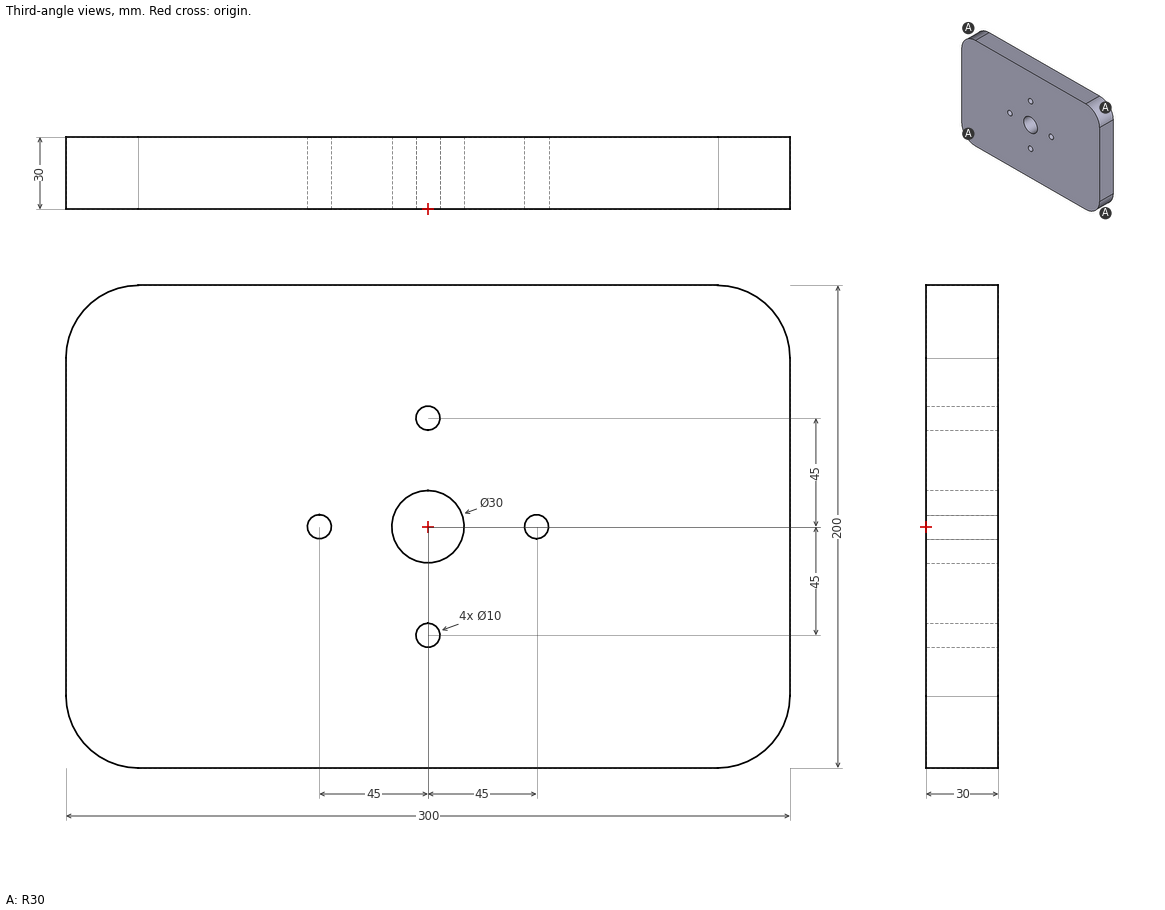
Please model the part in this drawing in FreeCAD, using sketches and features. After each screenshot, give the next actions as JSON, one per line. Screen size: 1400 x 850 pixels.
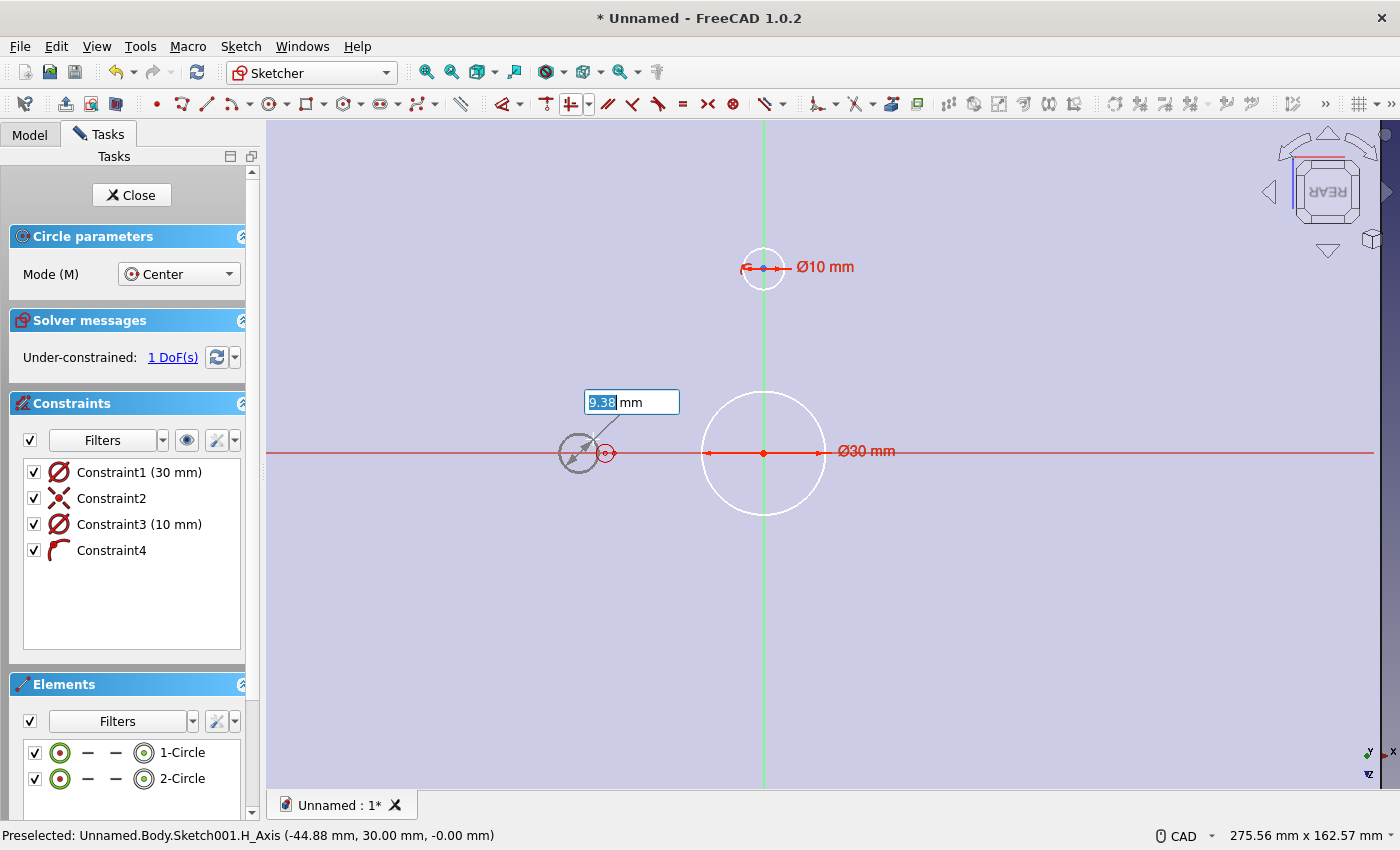
{"action": "type", "text": "10"}
{"action": "key", "text": "Return"}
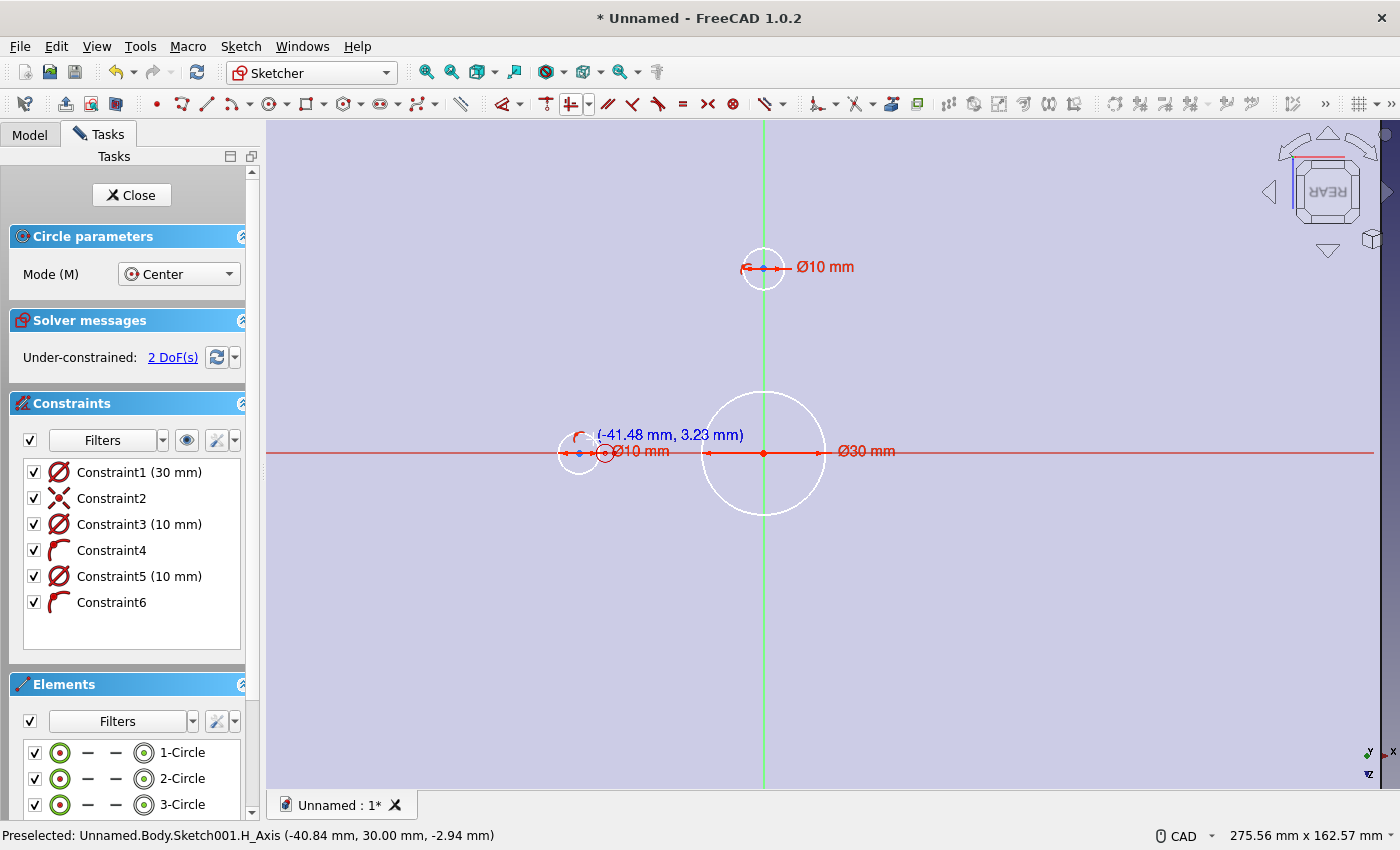
{"action": "left_click", "coordinate": [764, 638]}
{"action": "mouse_move", "coordinate": [778, 624]}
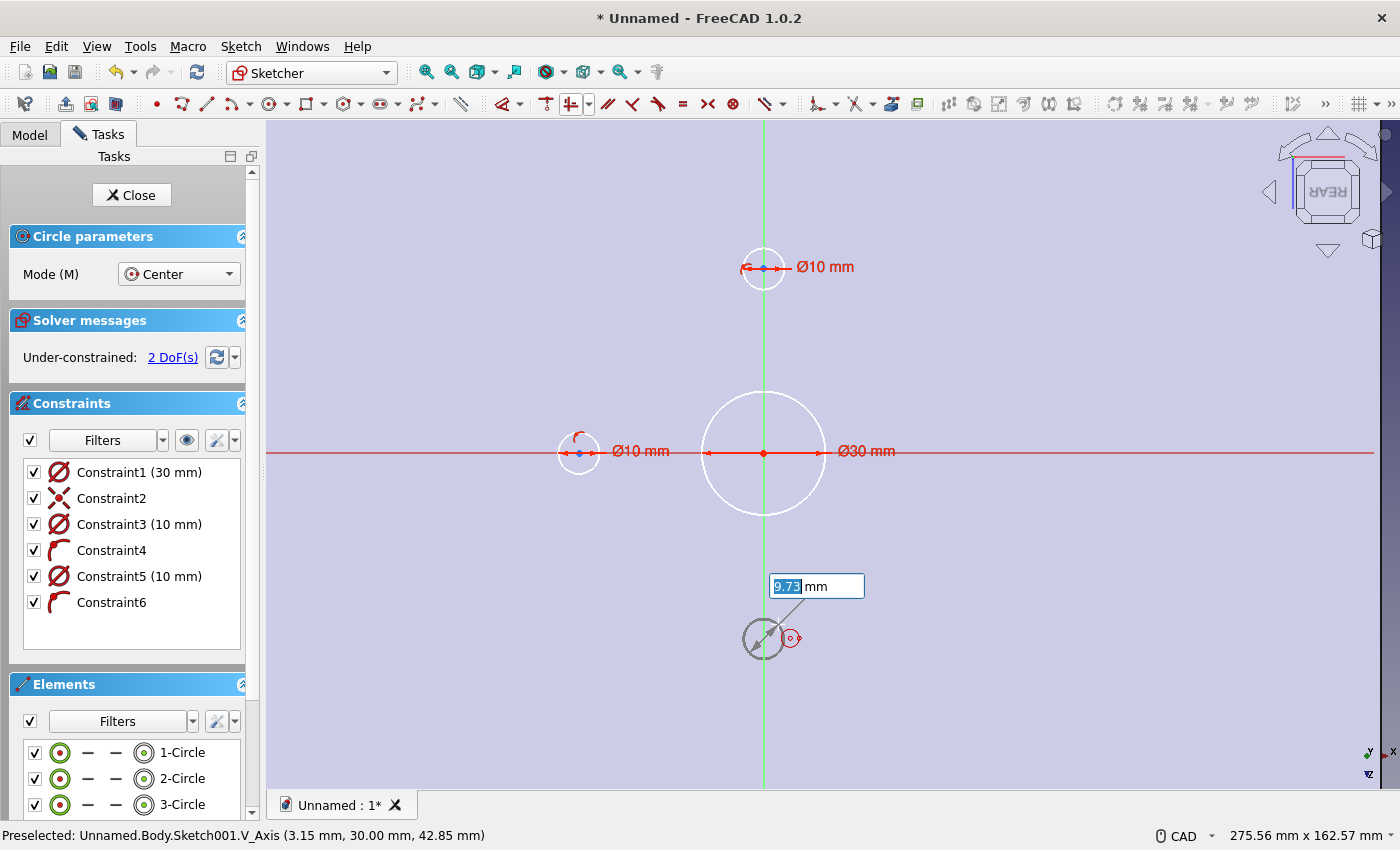
{"action": "type", "text": "10"}
{"action": "key", "text": "Return"}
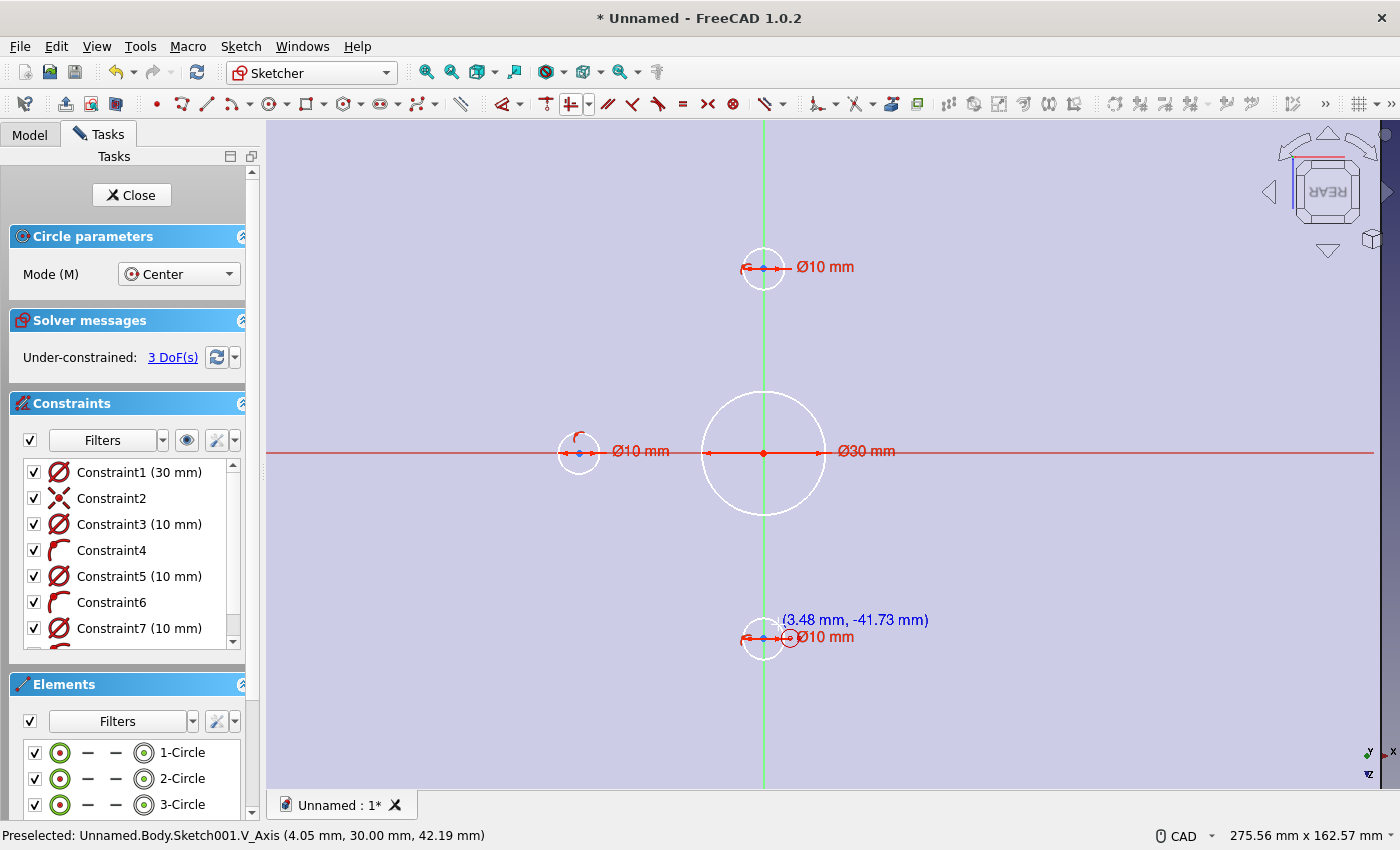
{"action": "left_click", "coordinate": [949, 453]}
{"action": "mouse_move", "coordinate": [963, 439]}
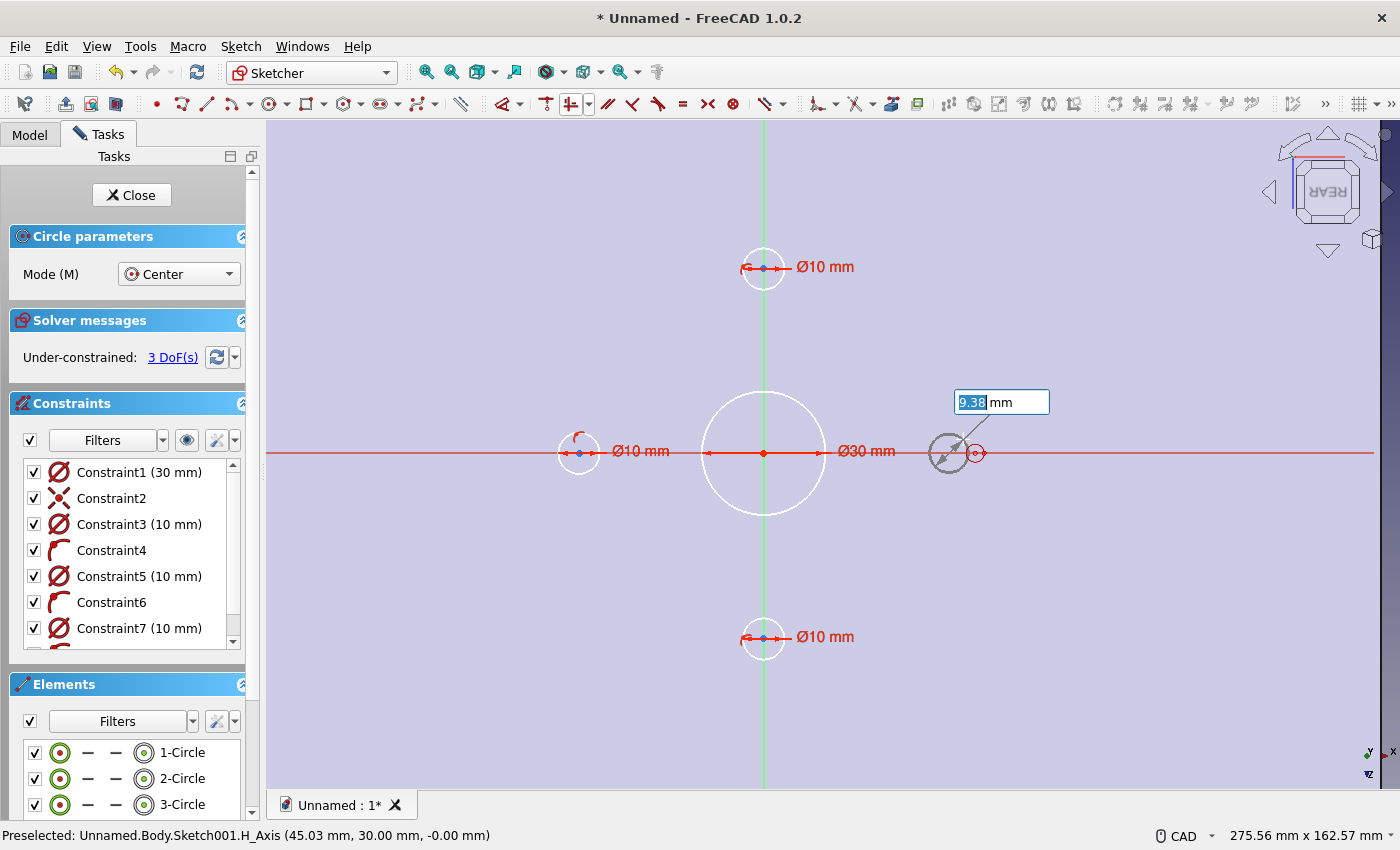
{"action": "type", "text": "10"}
{"action": "key", "text": "Return"}
{"action": "key", "text": "Escape"}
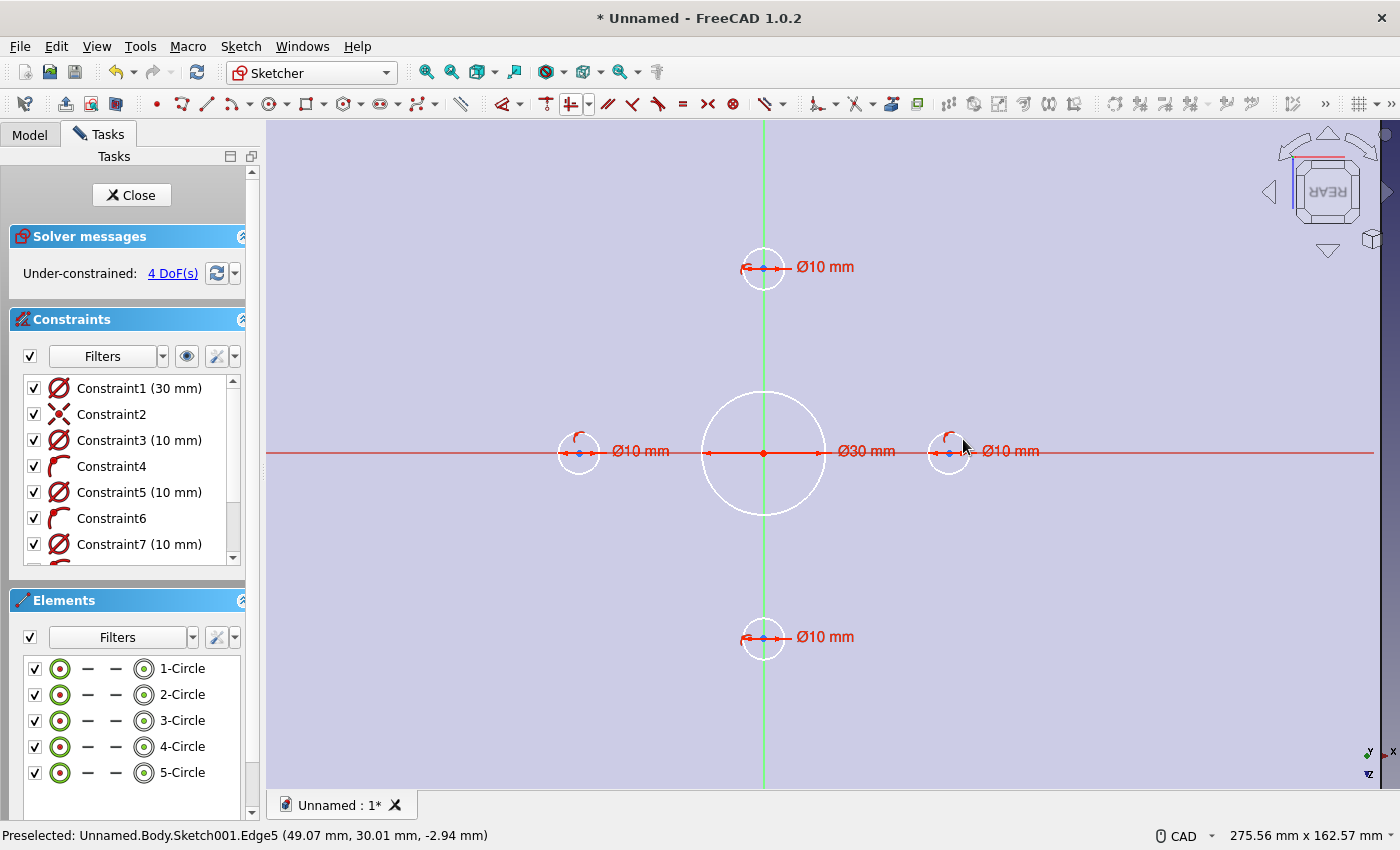
{"action": "left_click", "coordinate": [502, 104]}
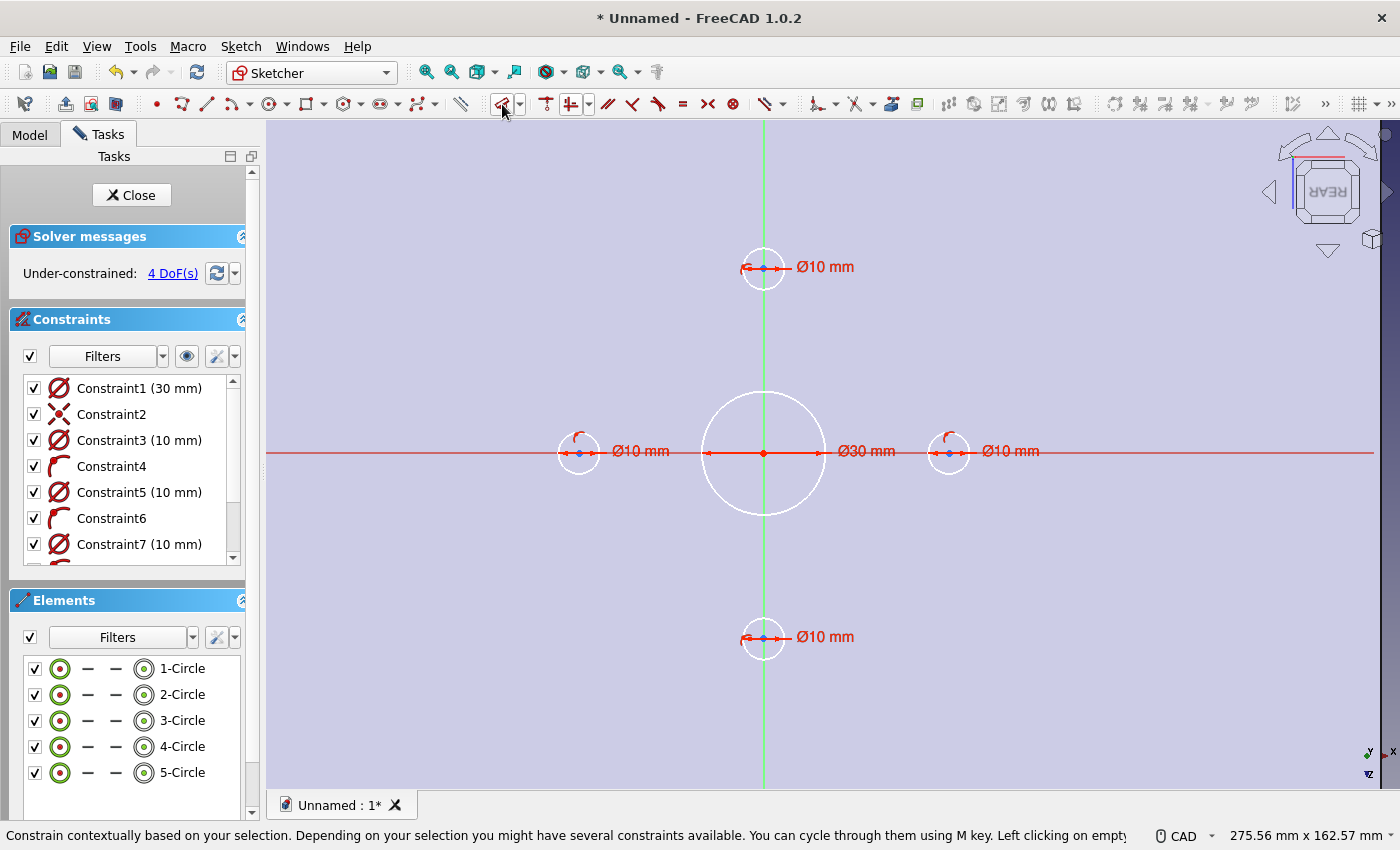
{"action": "left_click", "coordinate": [764, 269]}
{"action": "left_click", "coordinate": [798, 361]}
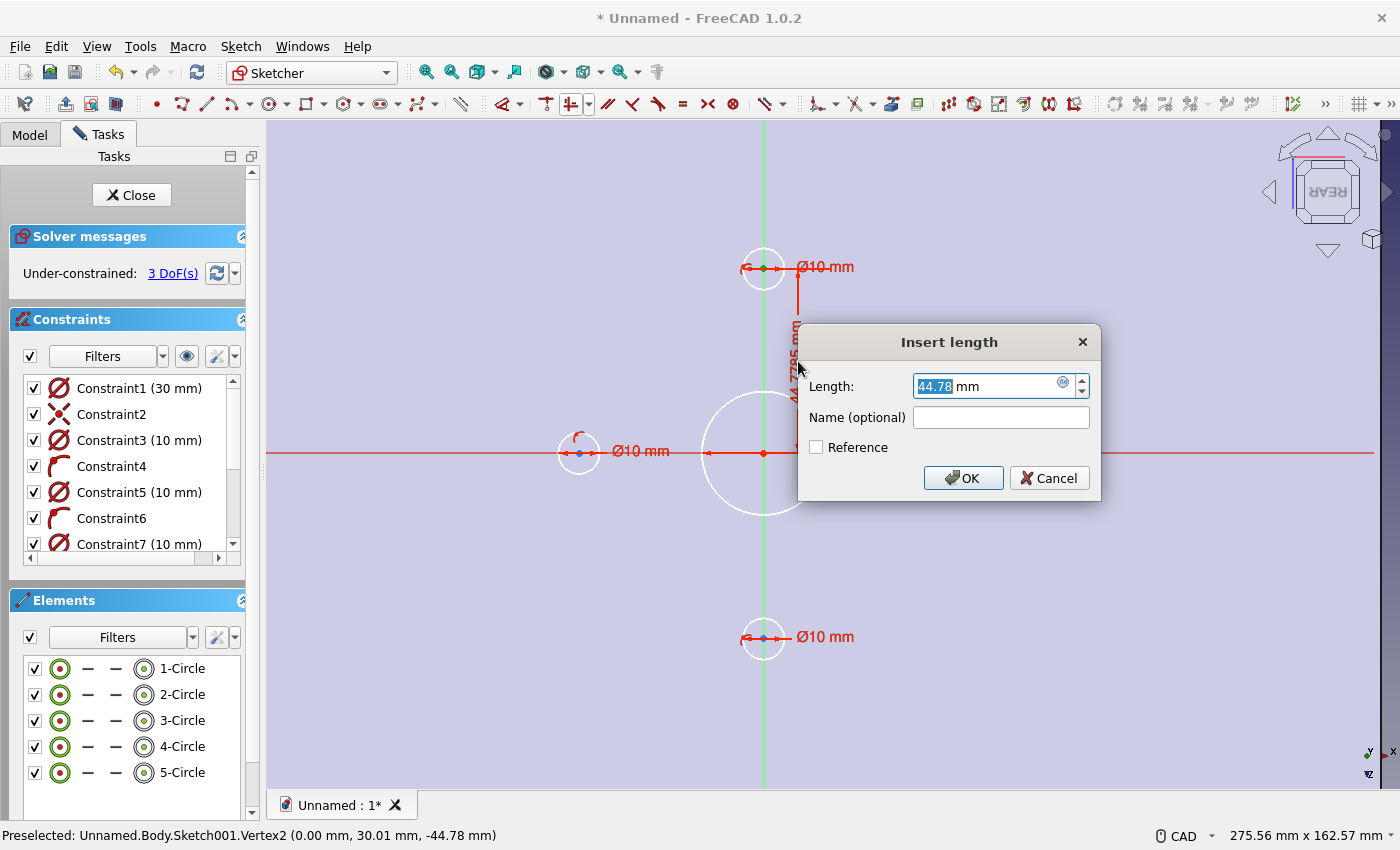
{"action": "type", "text": "45"}
{"action": "key", "text": "Return"}